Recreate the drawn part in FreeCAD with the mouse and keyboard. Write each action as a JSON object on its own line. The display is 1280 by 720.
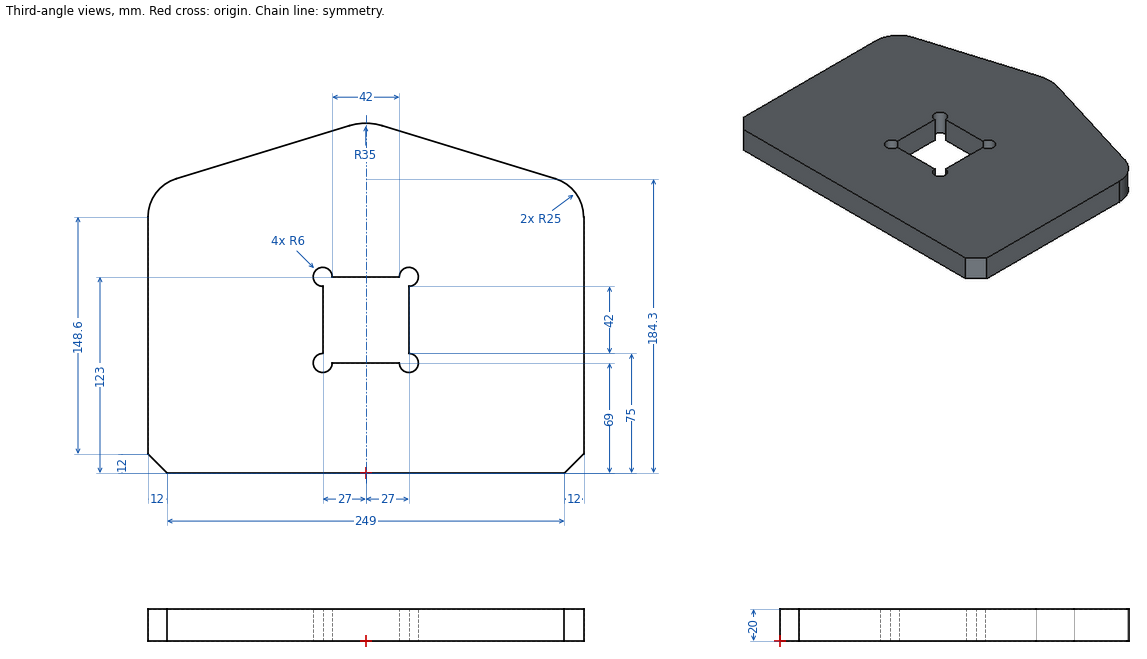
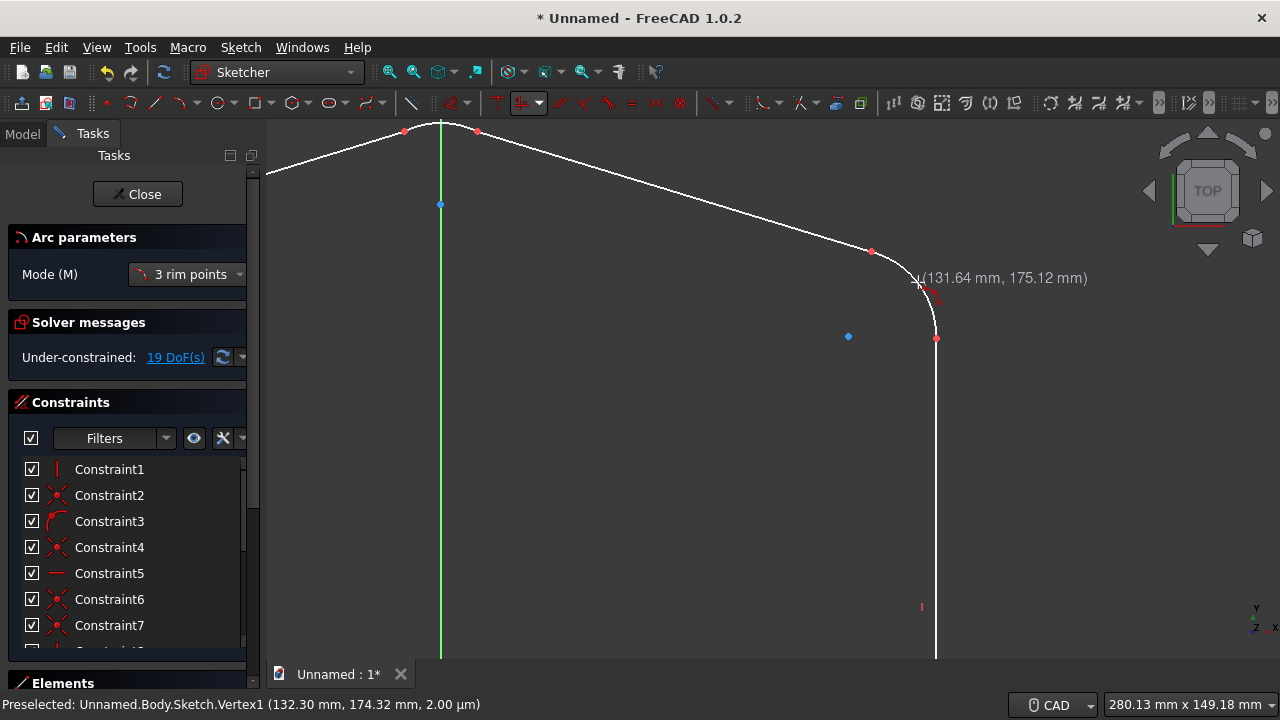
{"action": "left_click", "coordinate": [156, 104]}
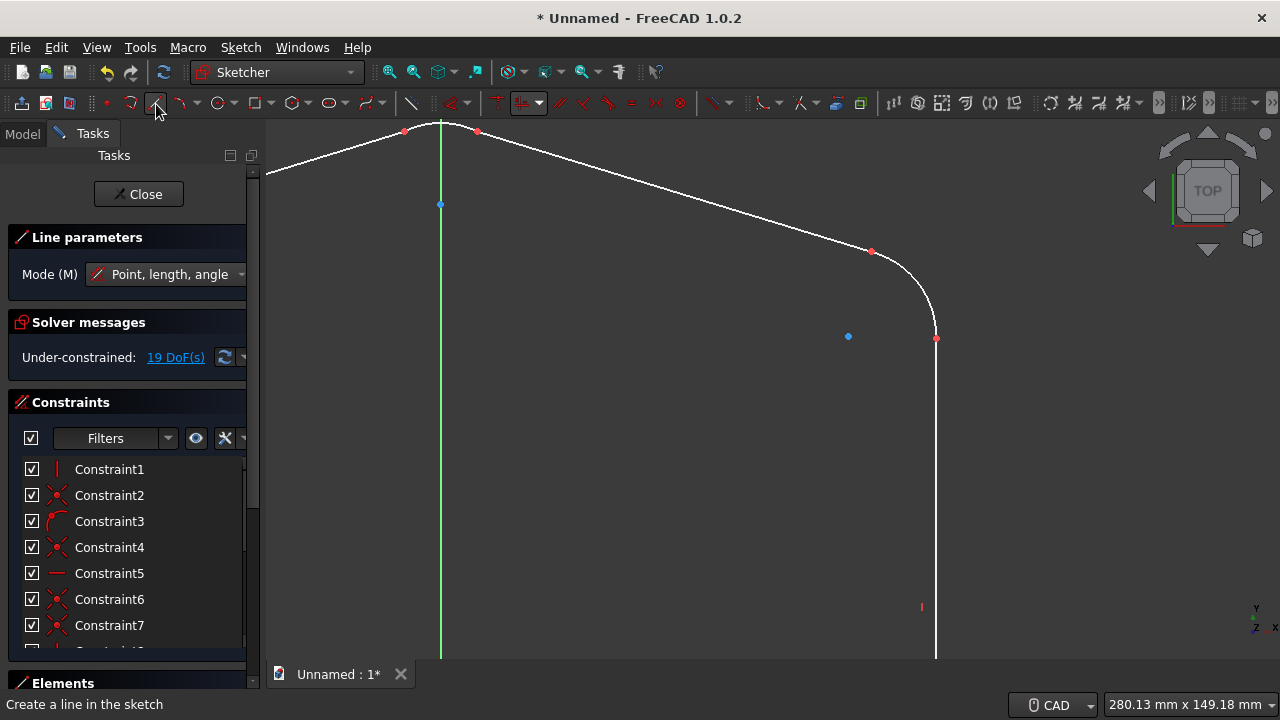
{"action": "left_click", "coordinate": [365, 472]}
{"action": "left_click", "coordinate": [518, 472]}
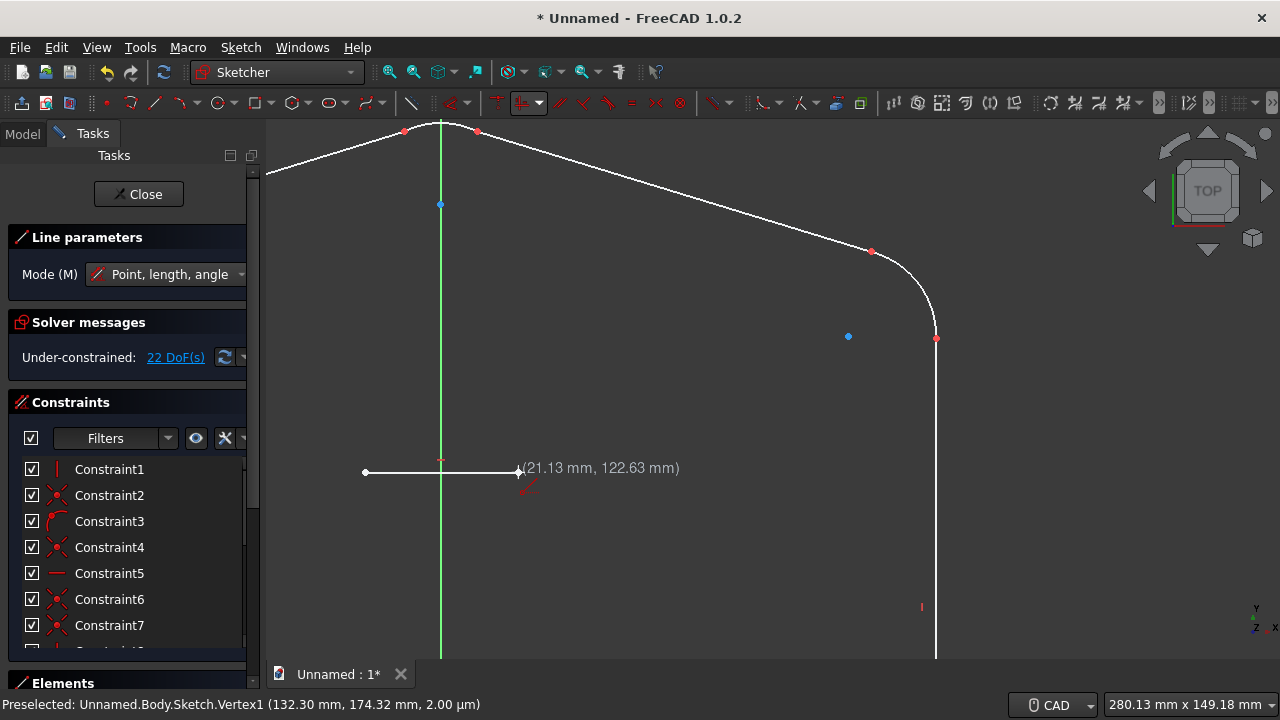
{"action": "left_click", "coordinate": [539, 493]}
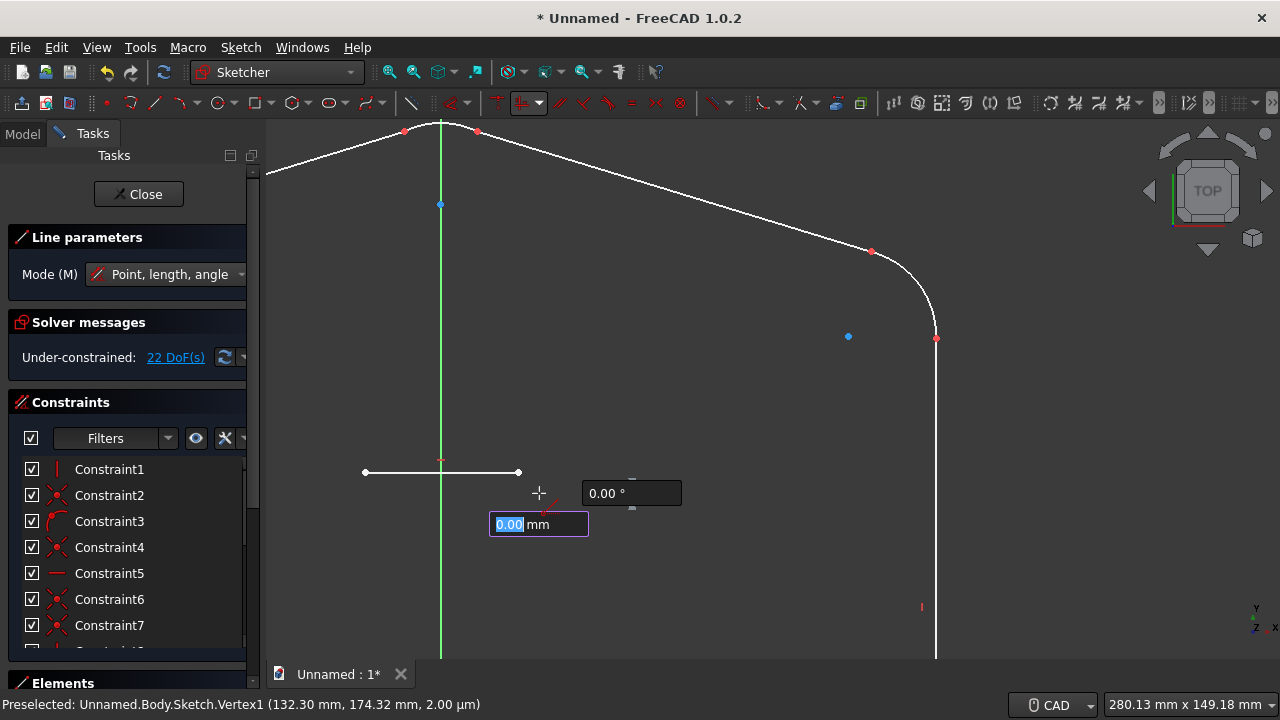
{"action": "scroll", "coordinate": [919, 282], "scroll_direction": "down", "scroll_amount": 4}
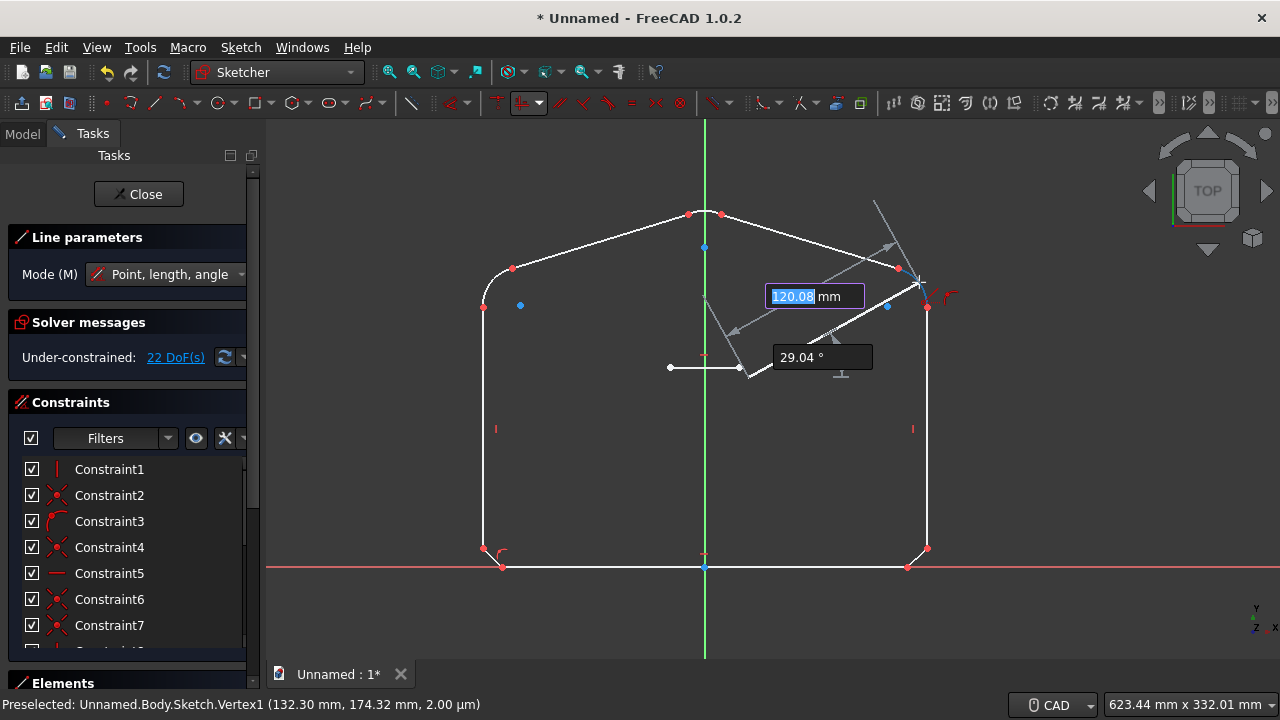
{"action": "left_click", "coordinate": [749, 445]}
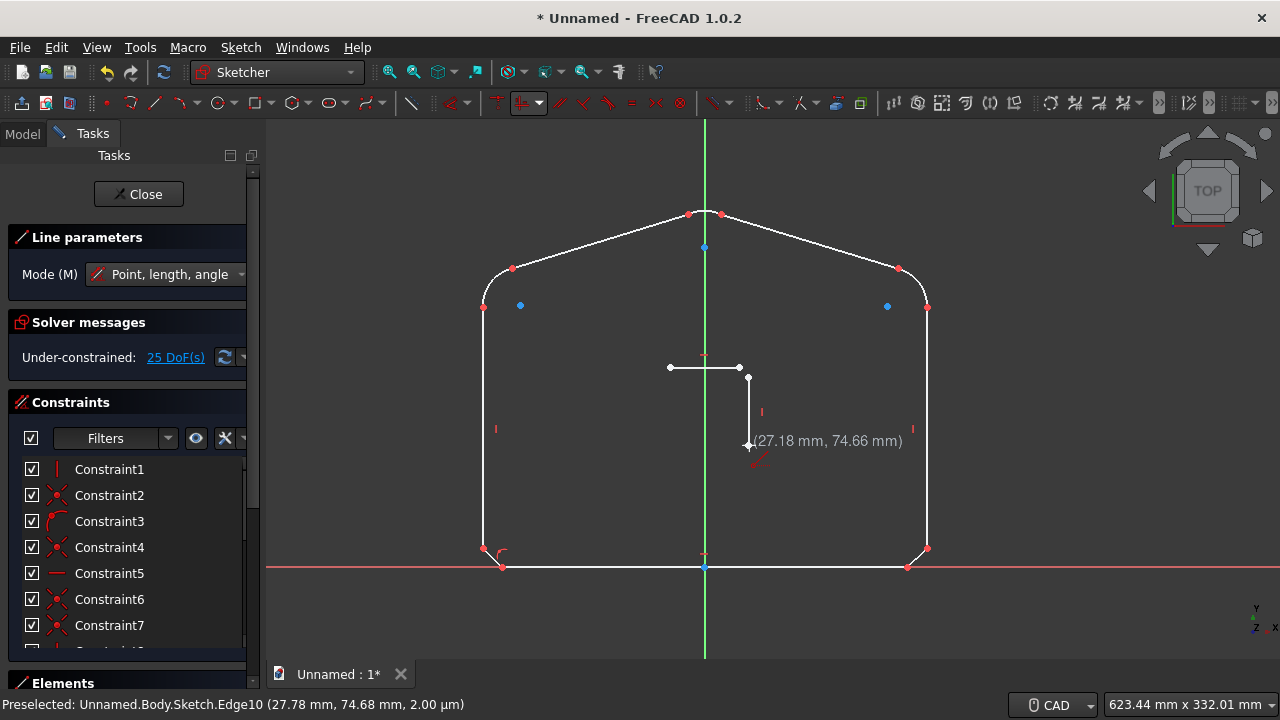
{"action": "left_click", "coordinate": [739, 455]}
{"action": "left_click", "coordinate": [671, 455]}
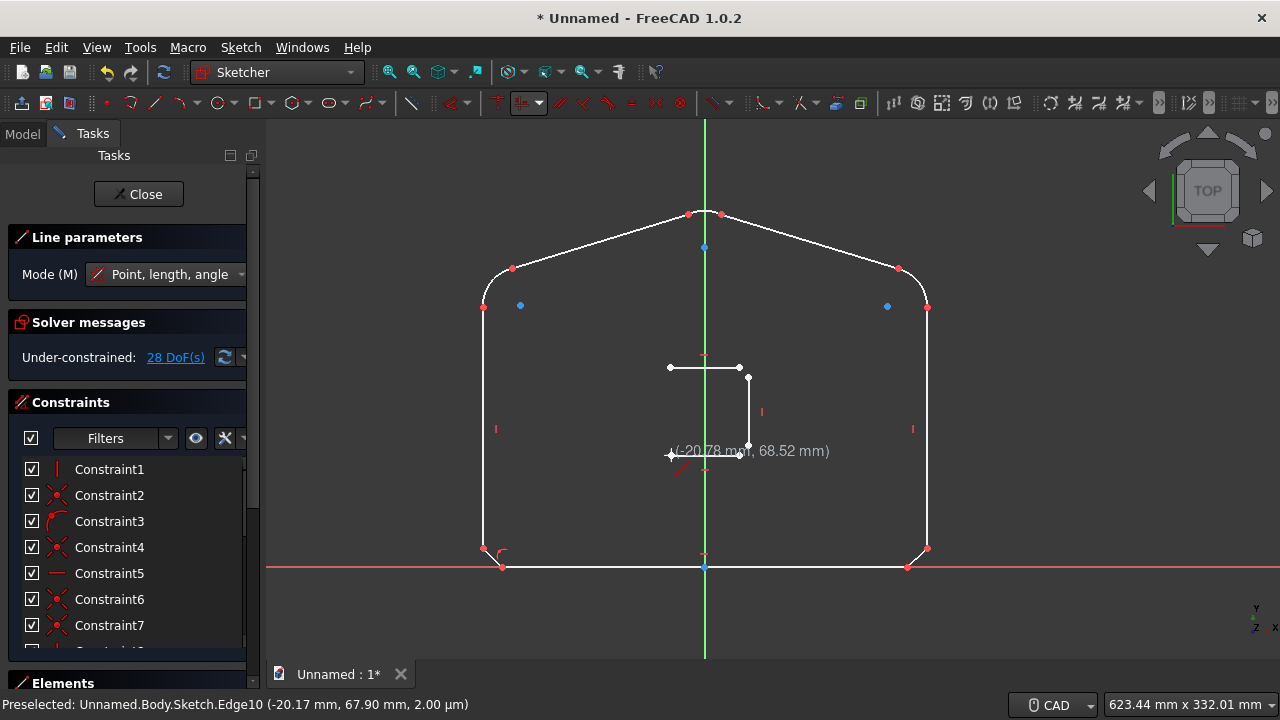
{"action": "left_click", "coordinate": [661, 445]}
{"action": "left_click", "coordinate": [661, 377]}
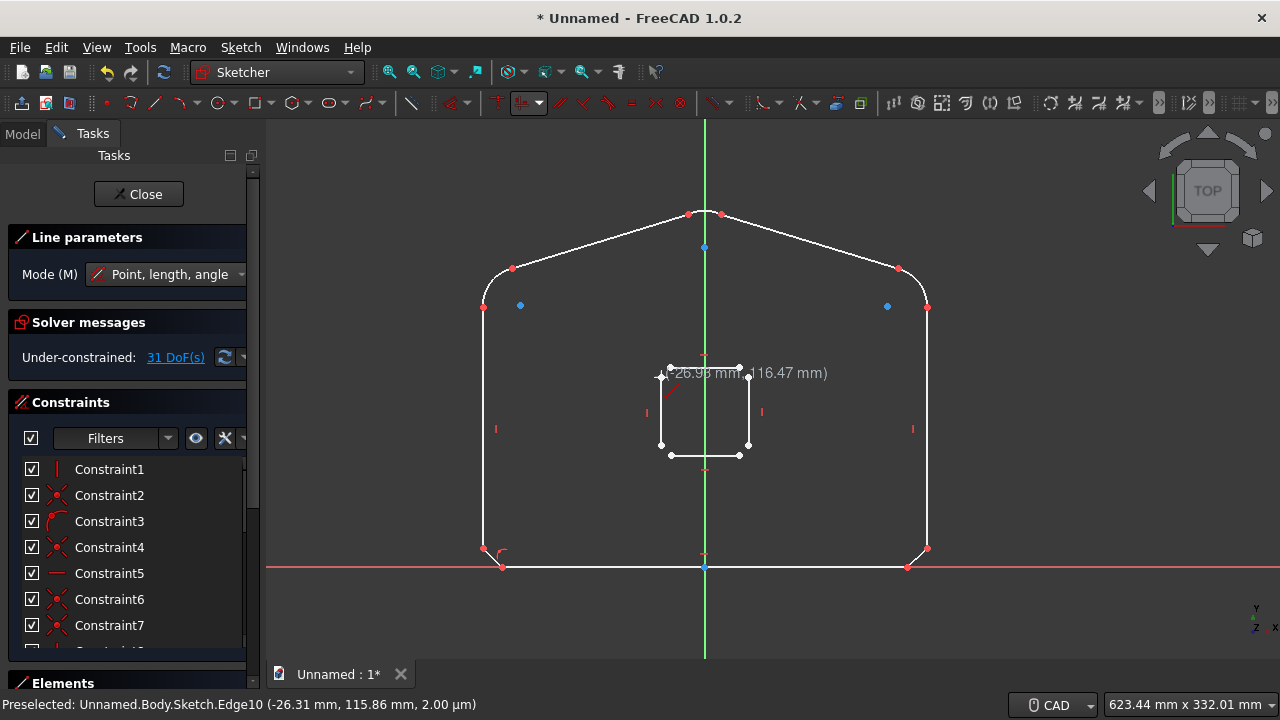
{"action": "left_click", "coordinate": [180, 104]}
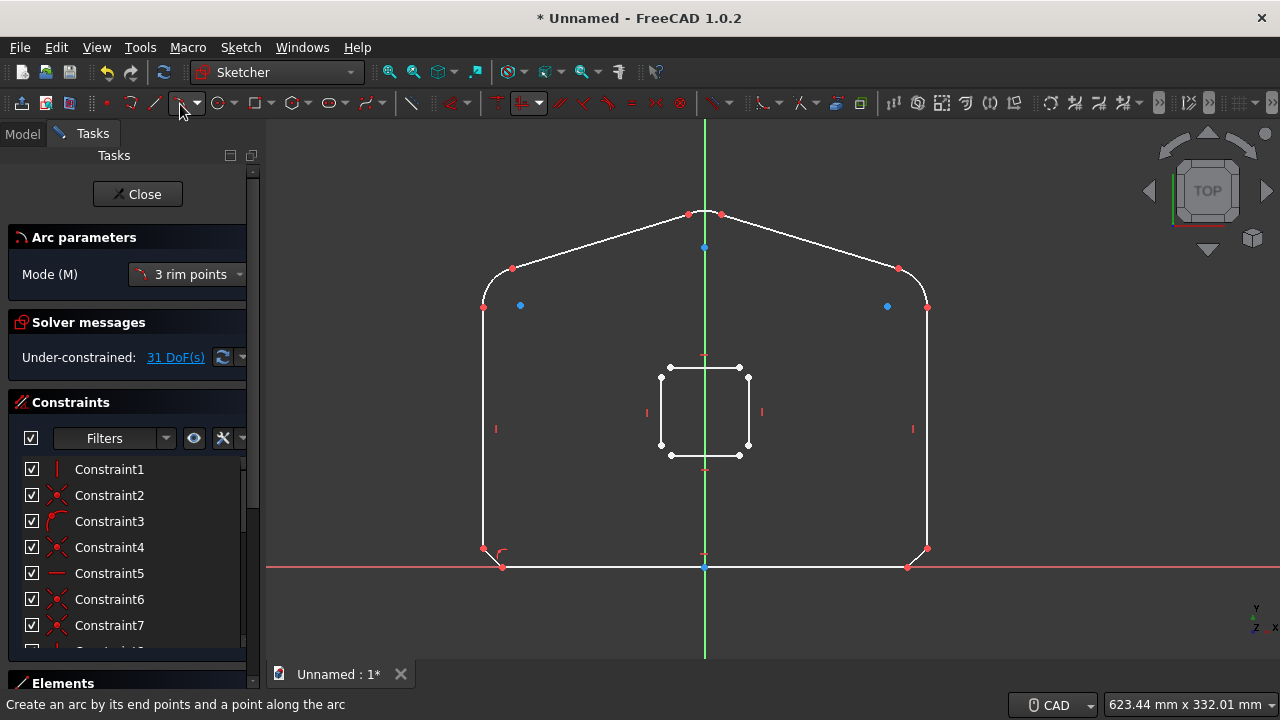
{"action": "left_click", "coordinate": [739, 368]}
{"action": "left_click", "coordinate": [749, 377]}
{"action": "left_click", "coordinate": [756, 360]}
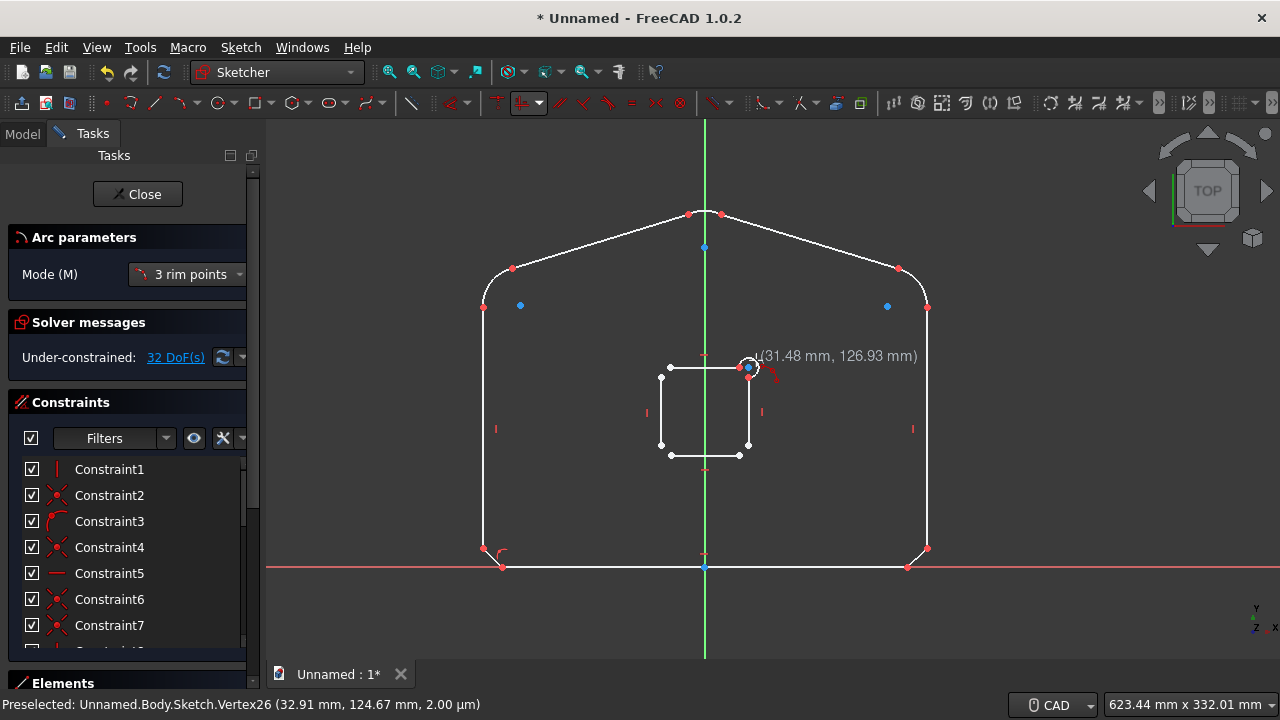
{"action": "left_click", "coordinate": [749, 446]}
{"action": "left_click", "coordinate": [739, 456]}
{"action": "left_click", "coordinate": [756, 462]}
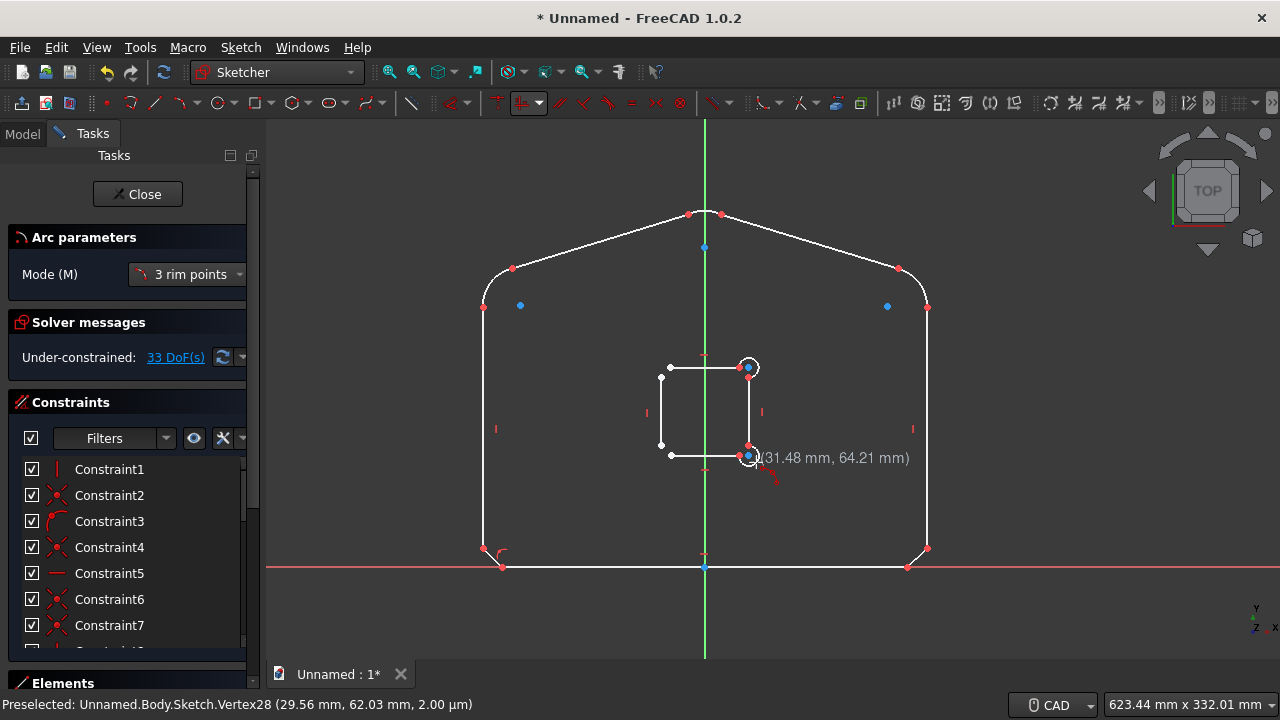
{"action": "left_click", "coordinate": [671, 456]}
{"action": "left_click", "coordinate": [661, 446]}
{"action": "left_click", "coordinate": [654, 462]}